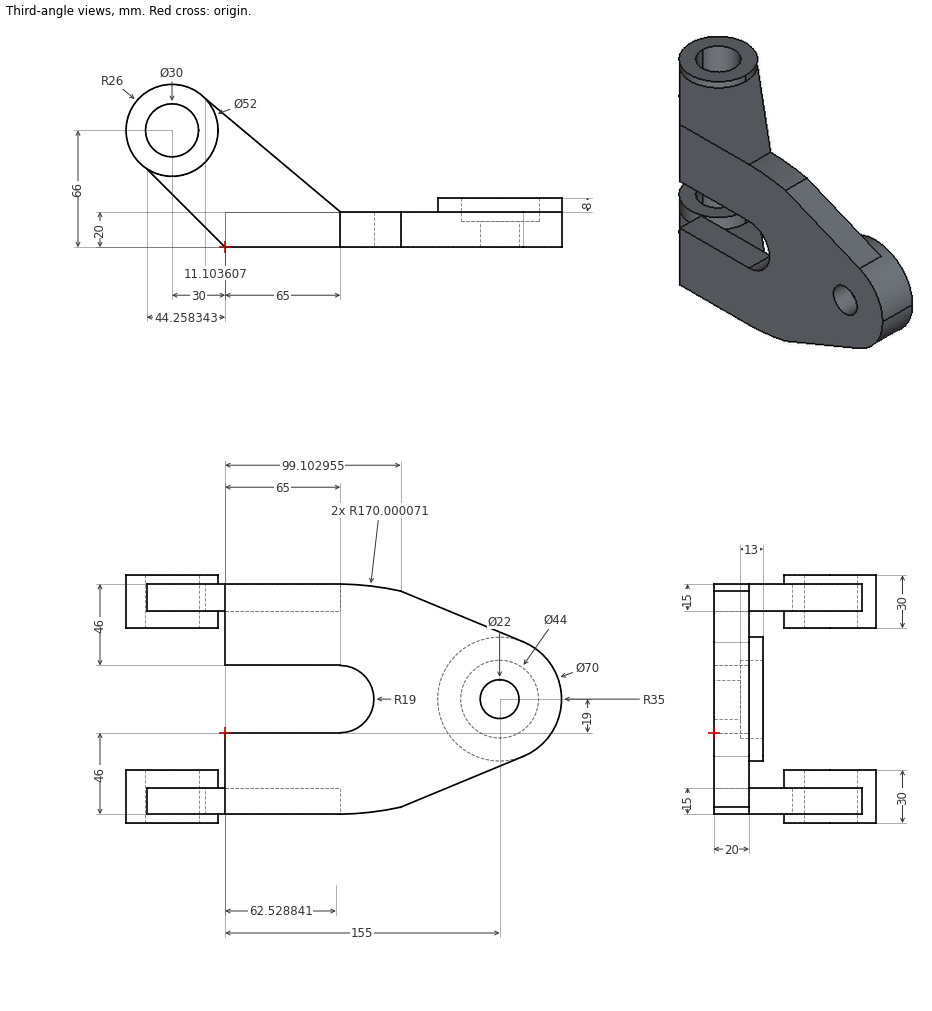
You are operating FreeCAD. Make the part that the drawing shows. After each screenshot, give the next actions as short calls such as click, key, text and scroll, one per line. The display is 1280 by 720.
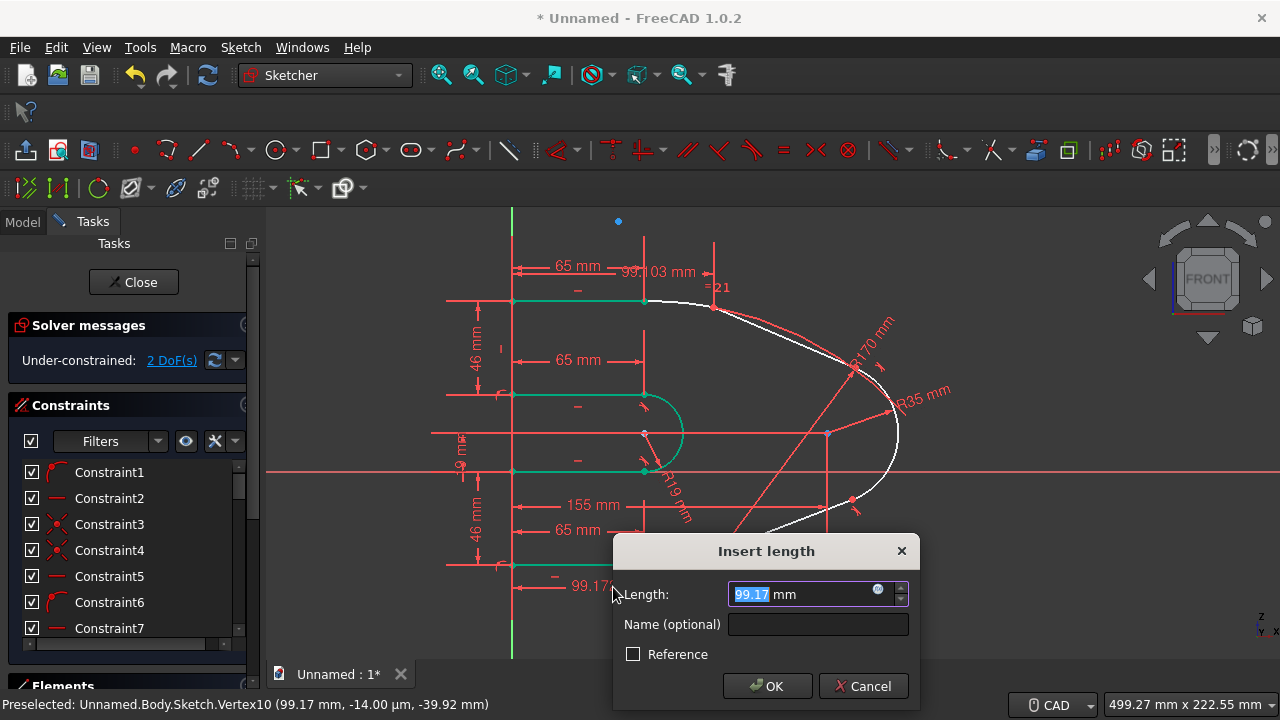
text(99.102955)
key(Return)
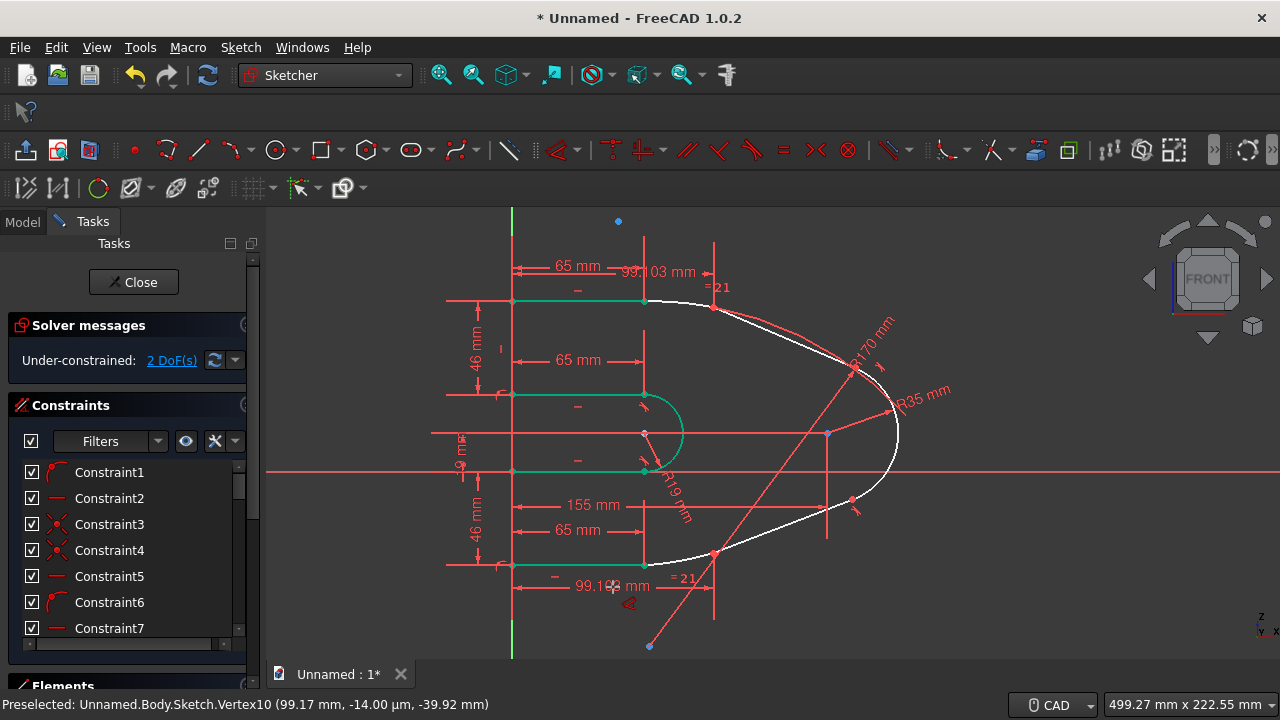
scroll(701, 248, down, 1)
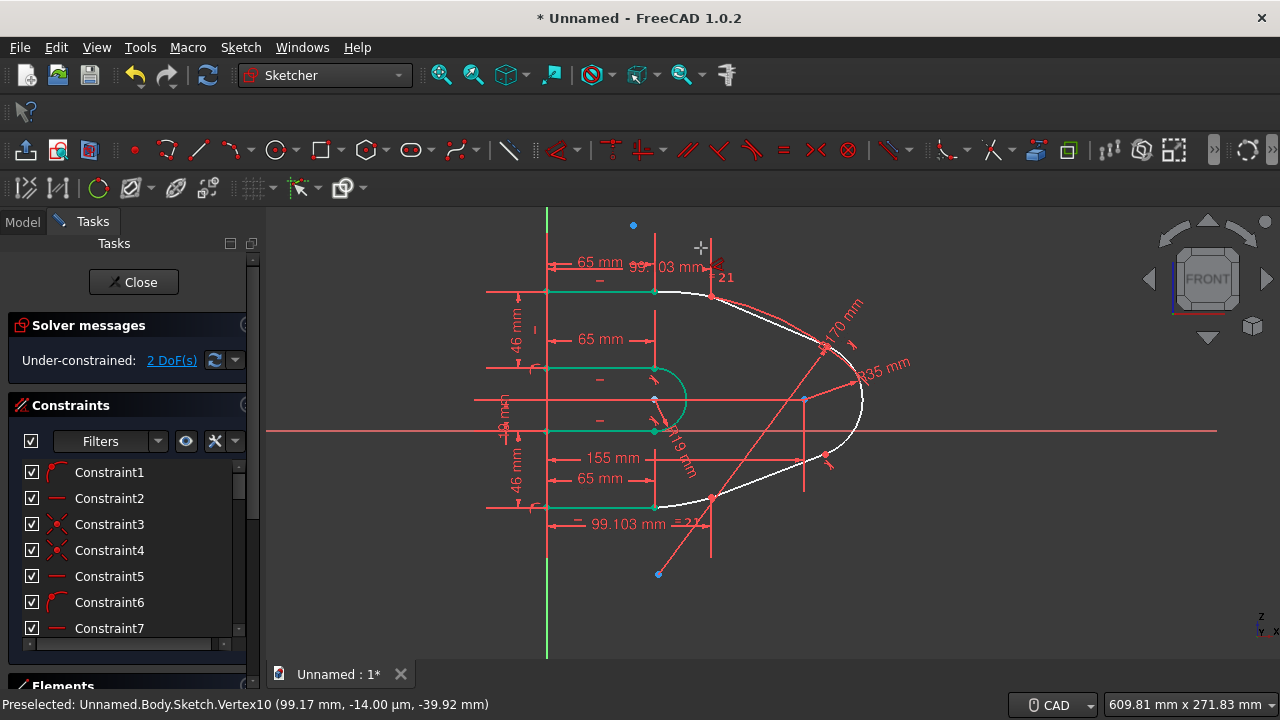
click(659, 574)
click(603, 608)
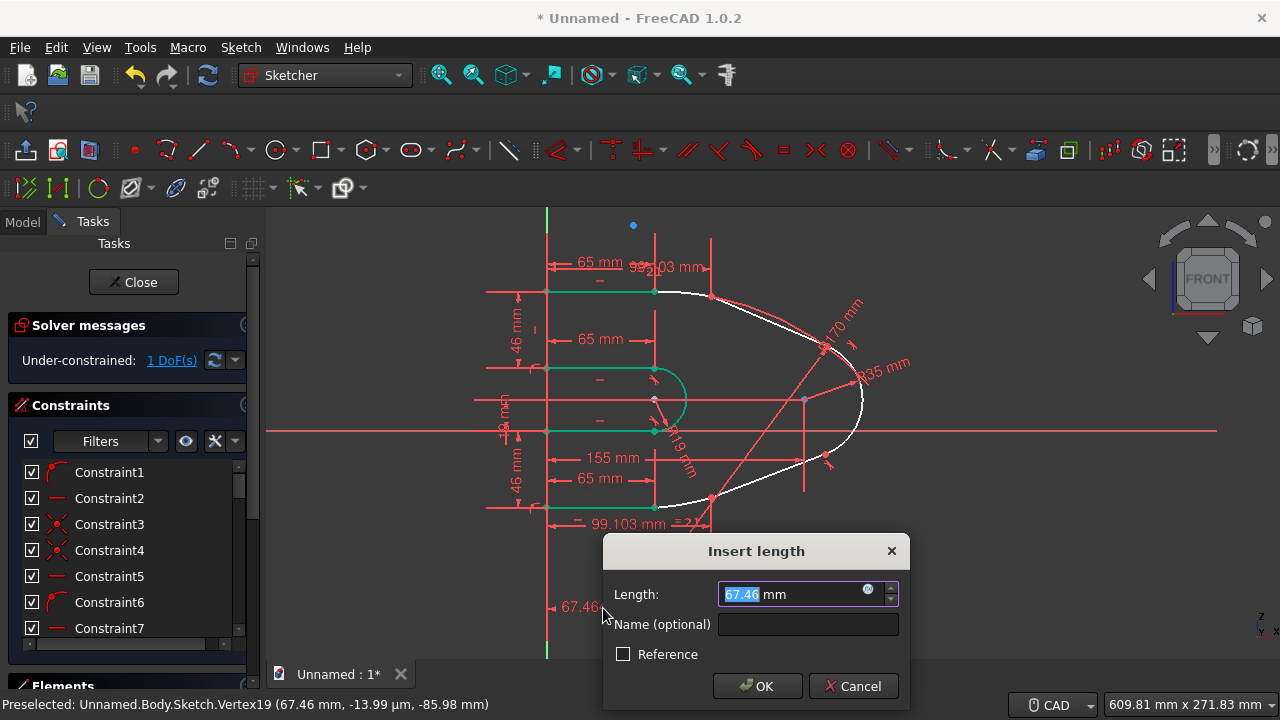
text(62.528841)
key(Return)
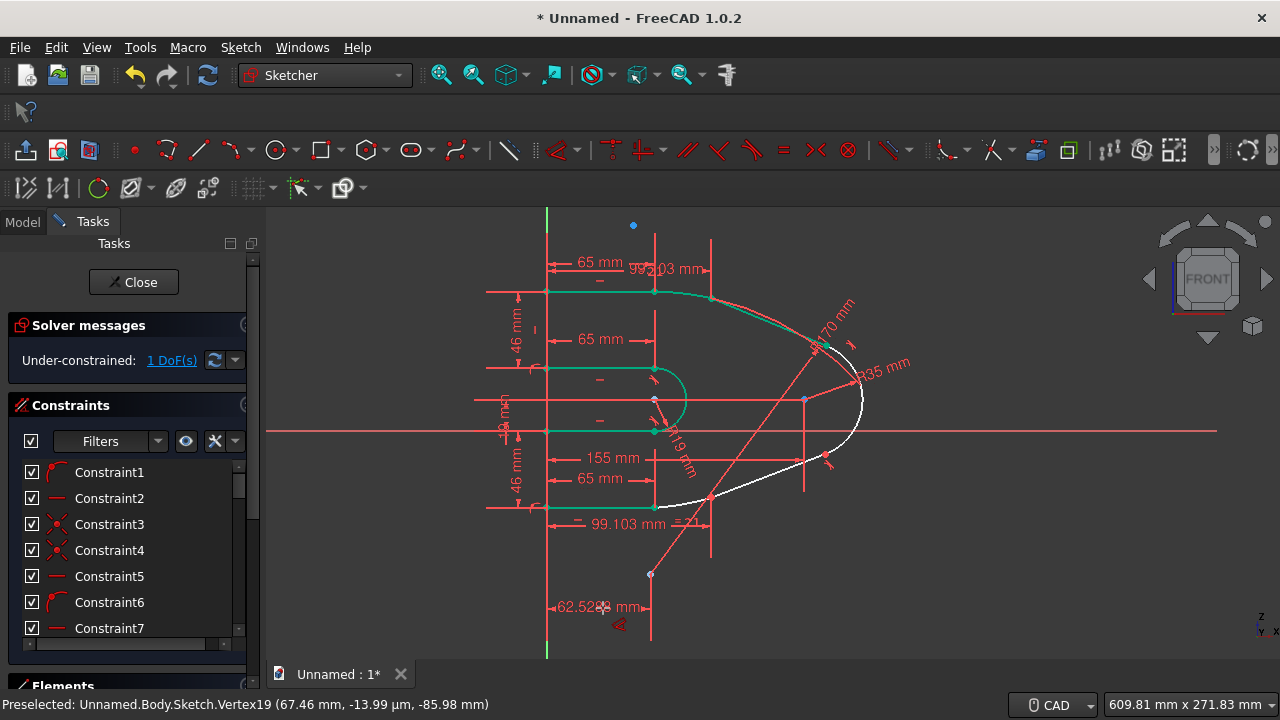
scroll(704, 631, down, 1)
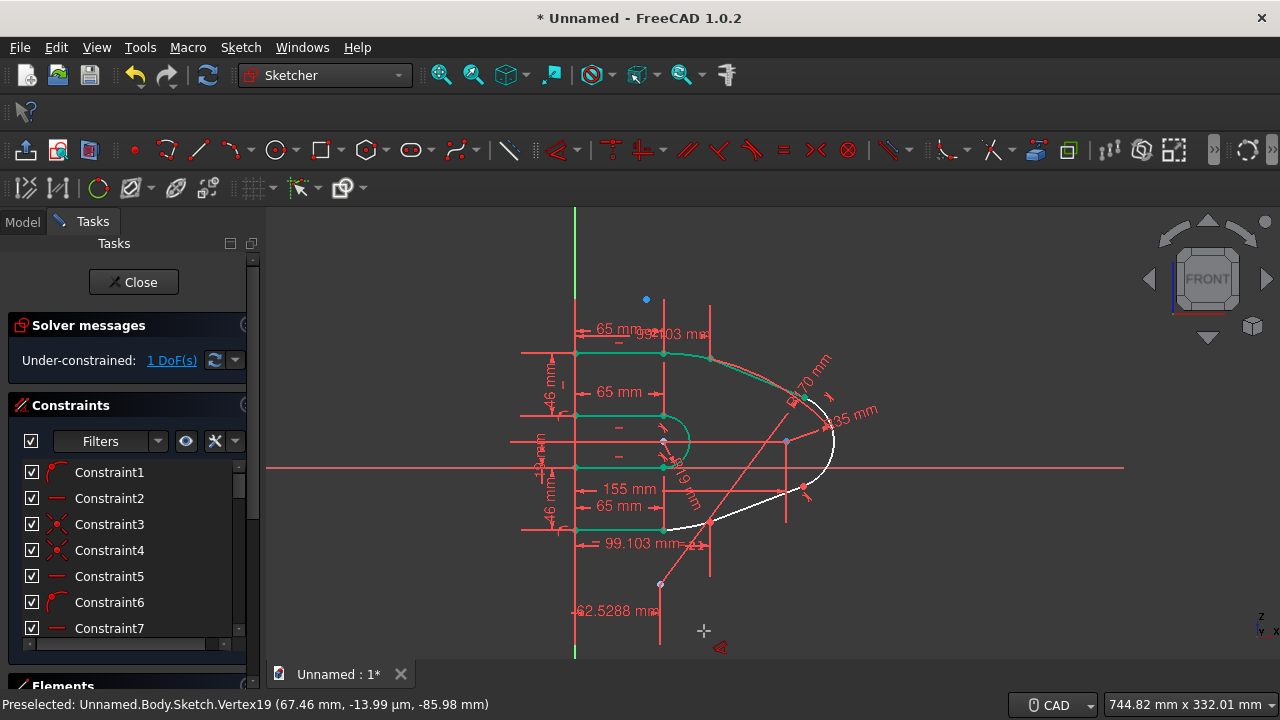
click(647, 300)
click(611, 266)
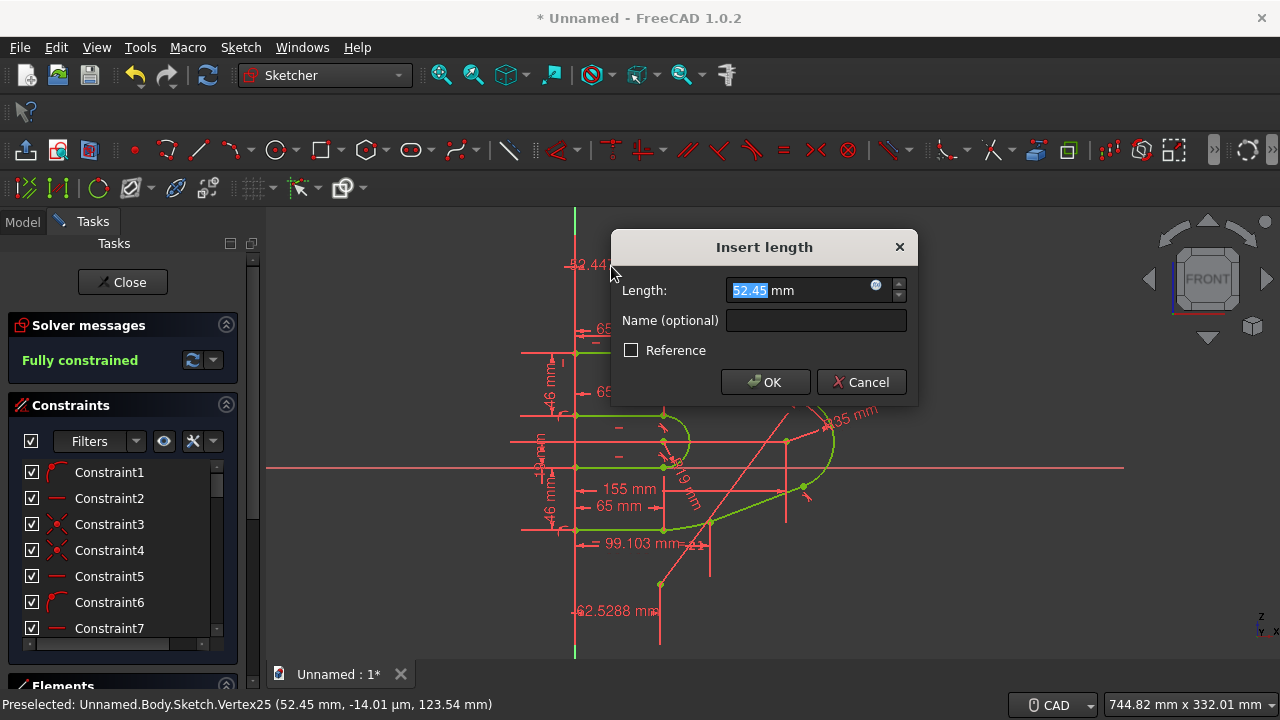
text(62.528841)
key(Return)
key(Escape)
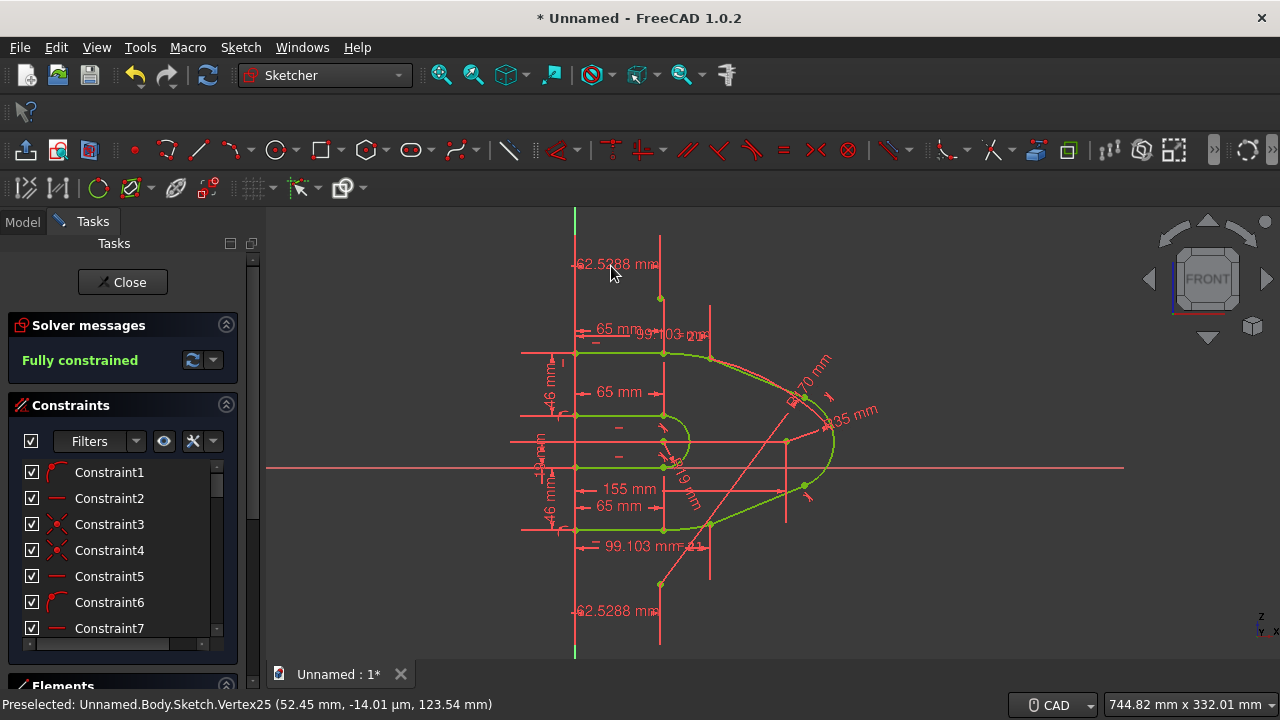
click(123, 282)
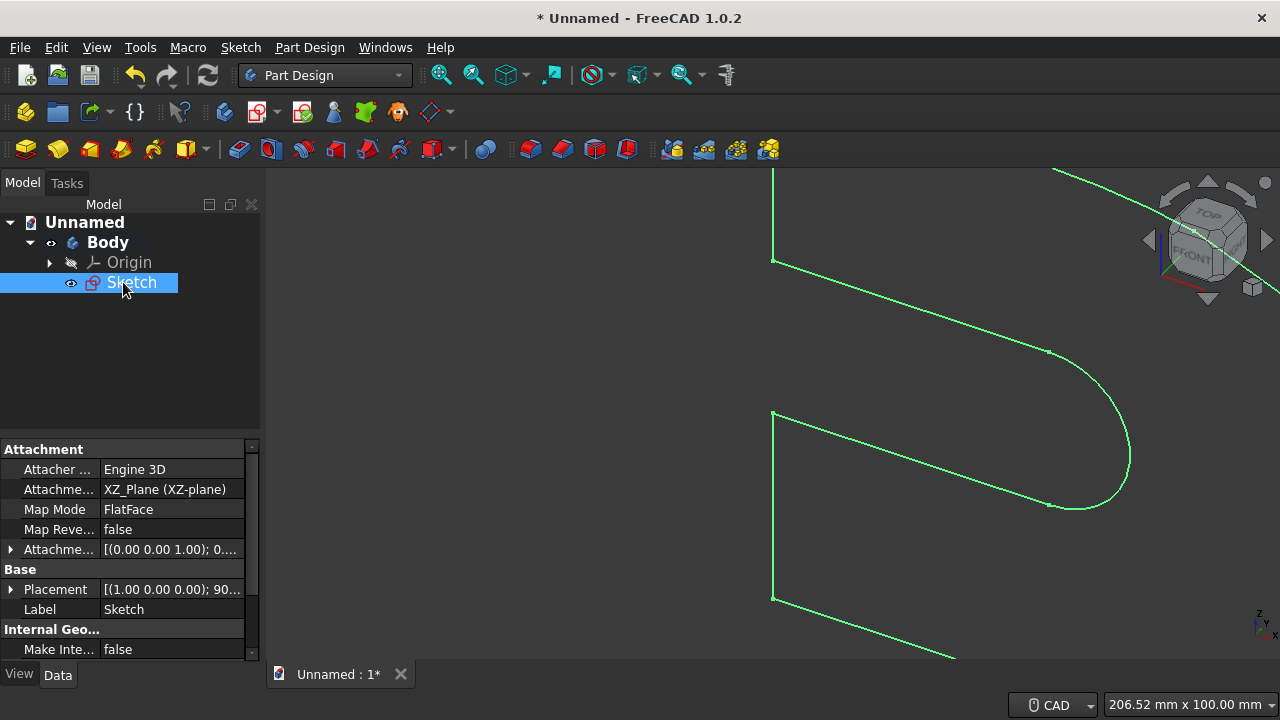
click(26, 150)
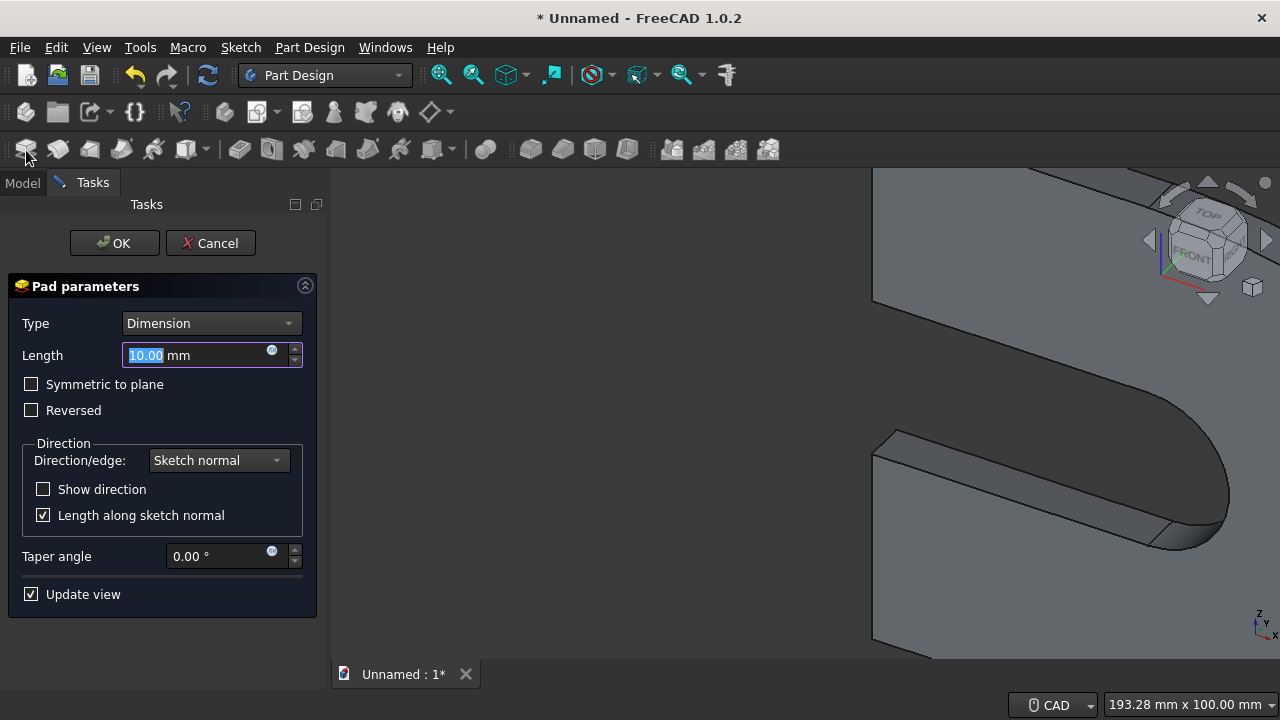
text(20)
key(Tab)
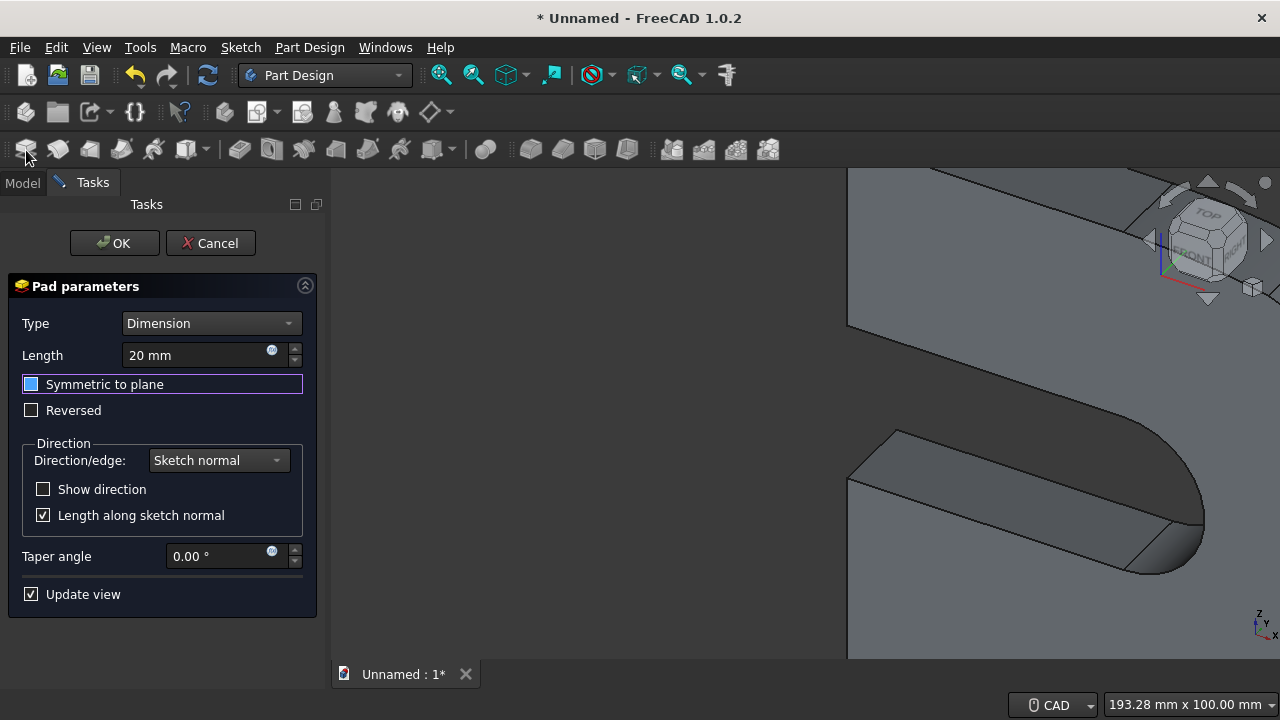
click(30, 410)